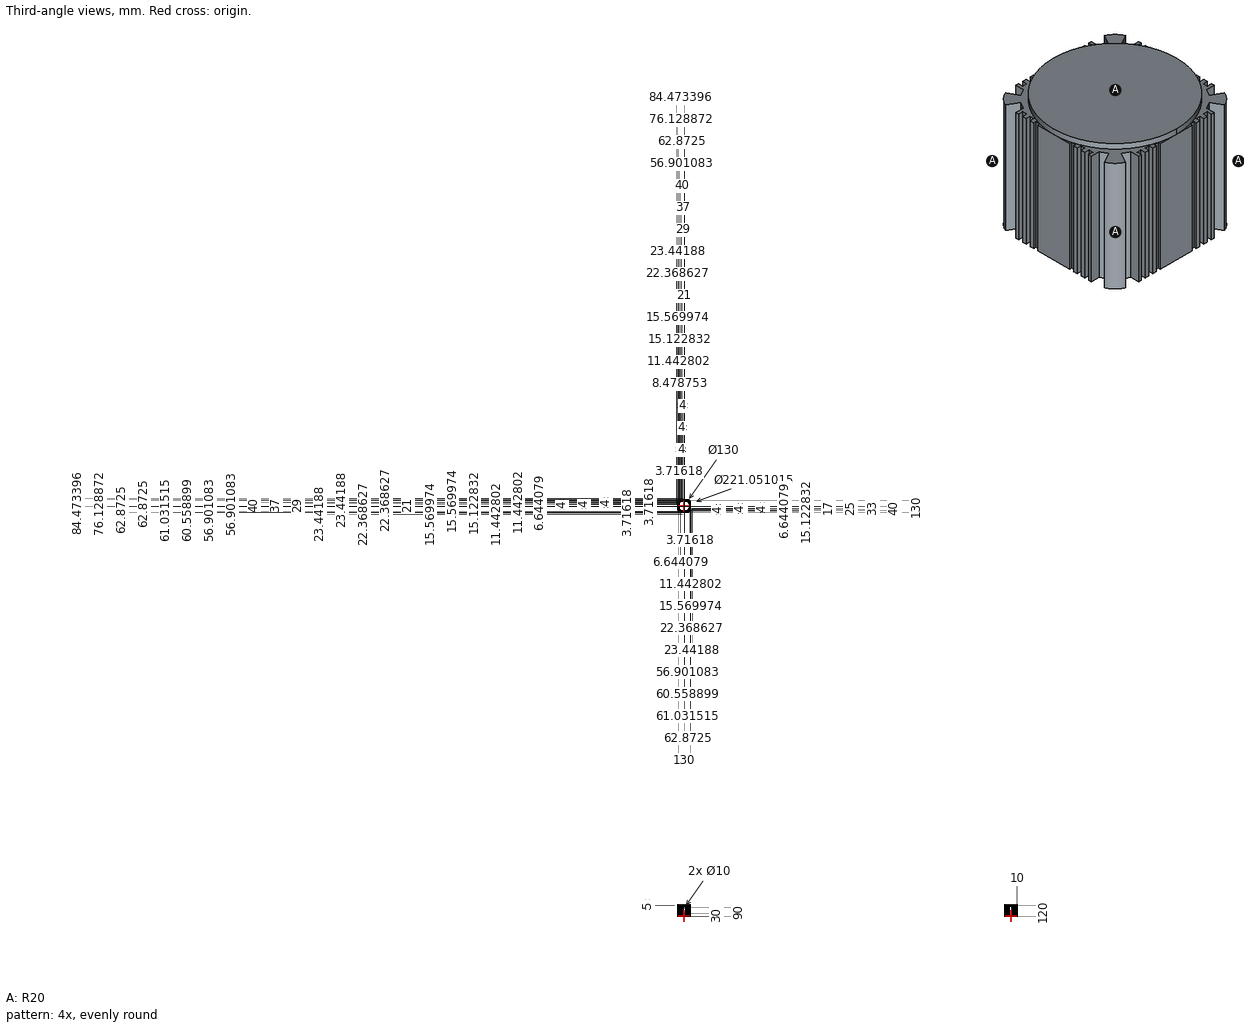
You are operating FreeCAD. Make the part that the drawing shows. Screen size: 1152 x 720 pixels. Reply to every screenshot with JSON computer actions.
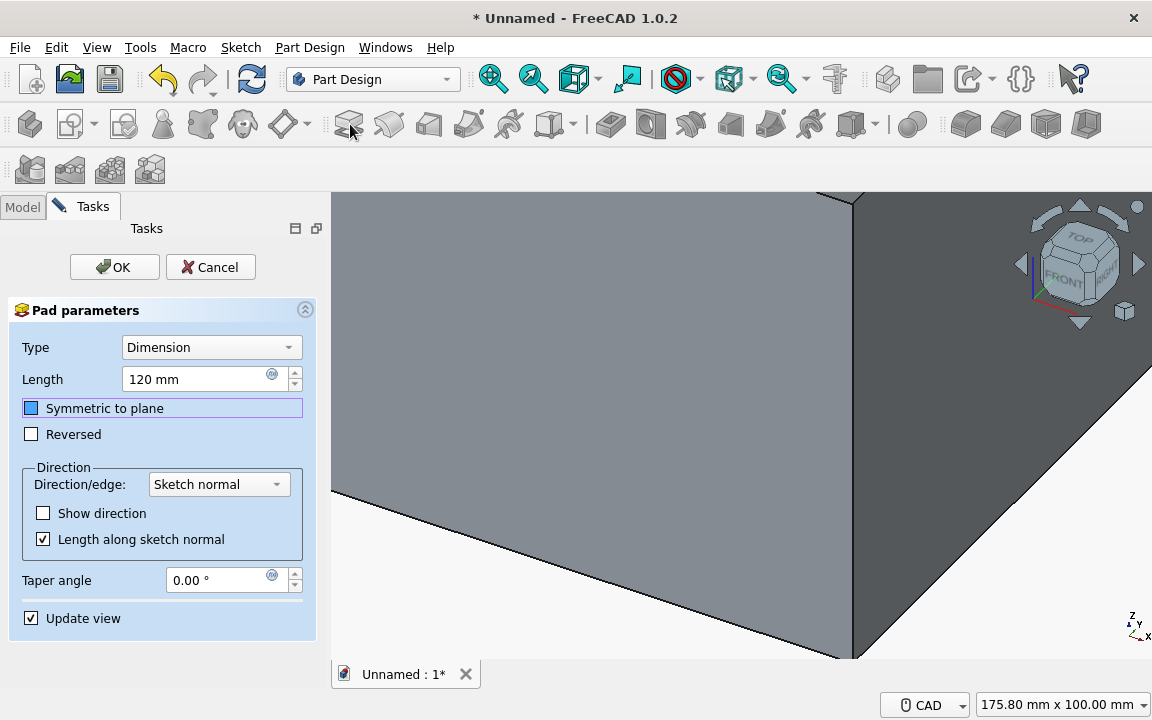
{"action": "left_click", "coordinate": [115, 267]}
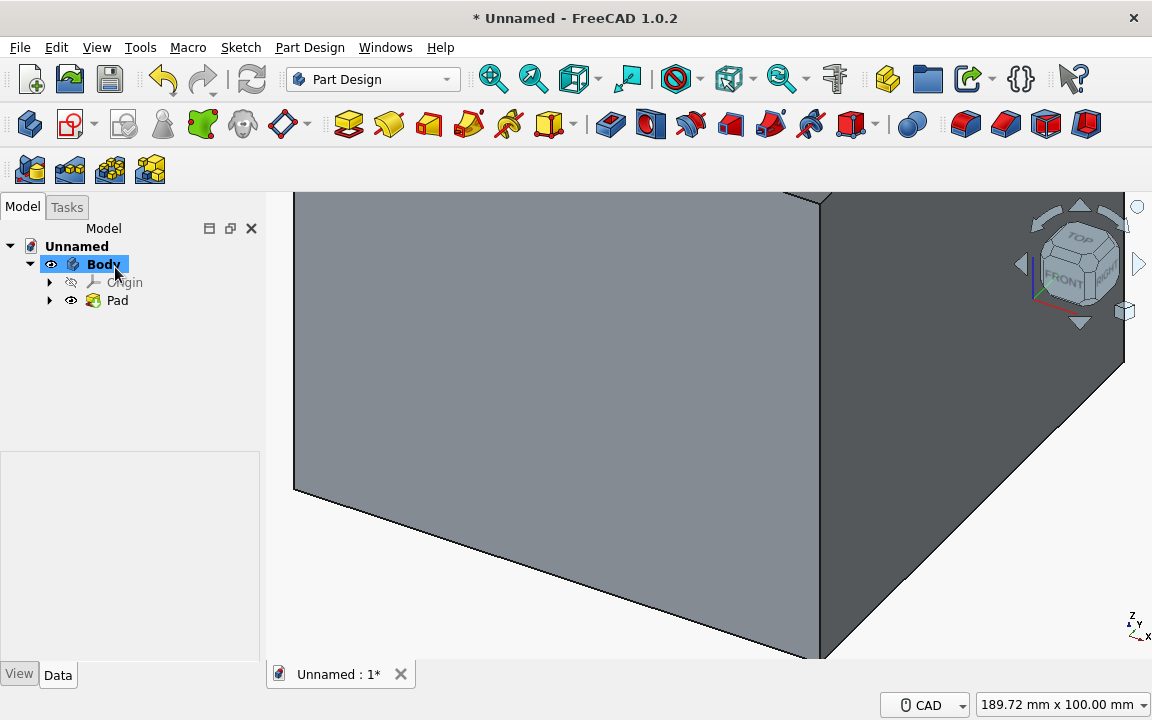
{"action": "left_click", "coordinate": [494, 80]}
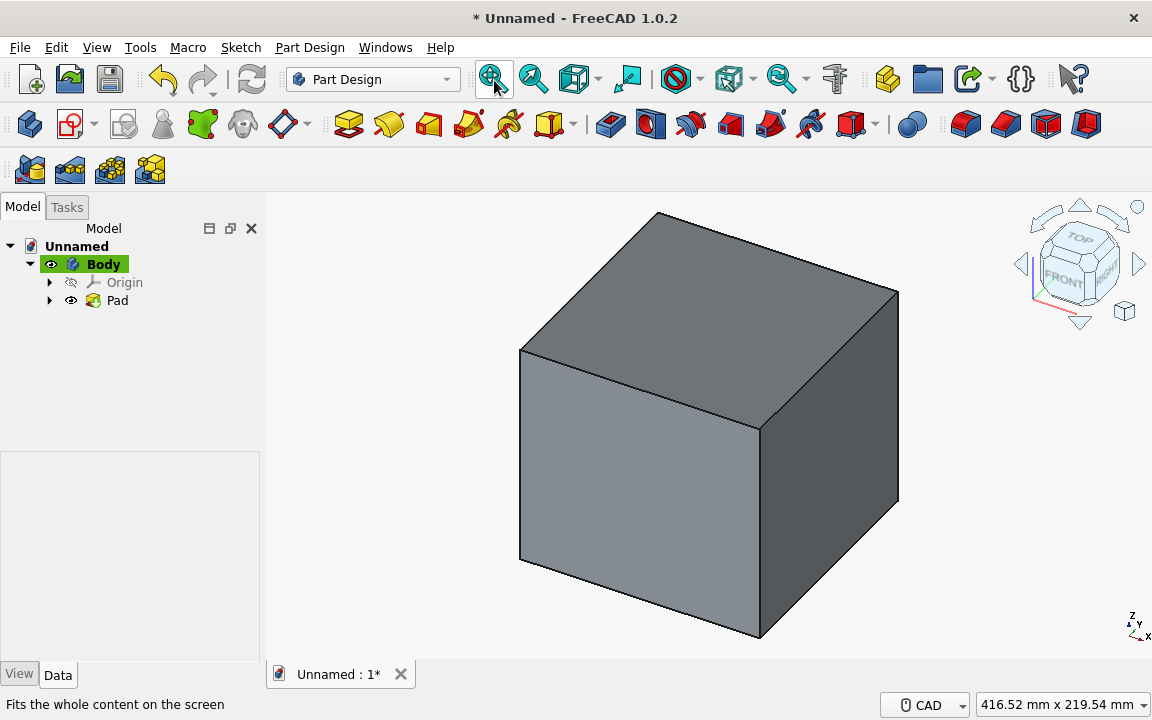
{"action": "left_click", "coordinate": [709, 320]}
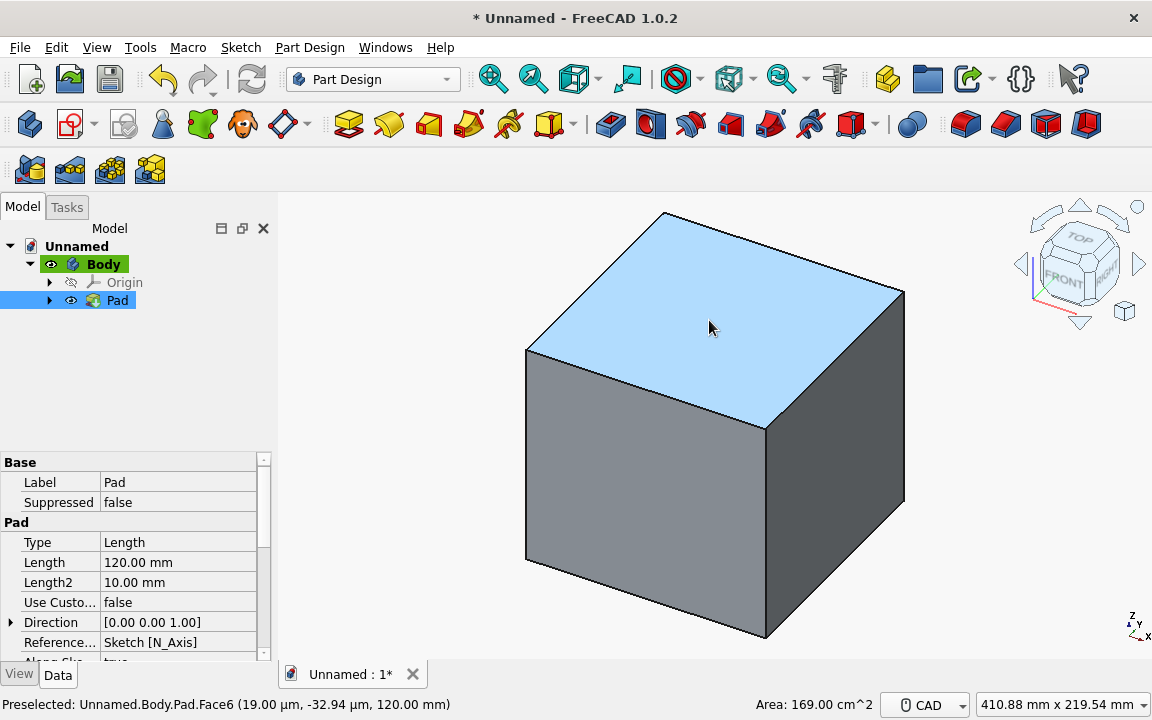
{"action": "left_click", "coordinate": [70, 124]}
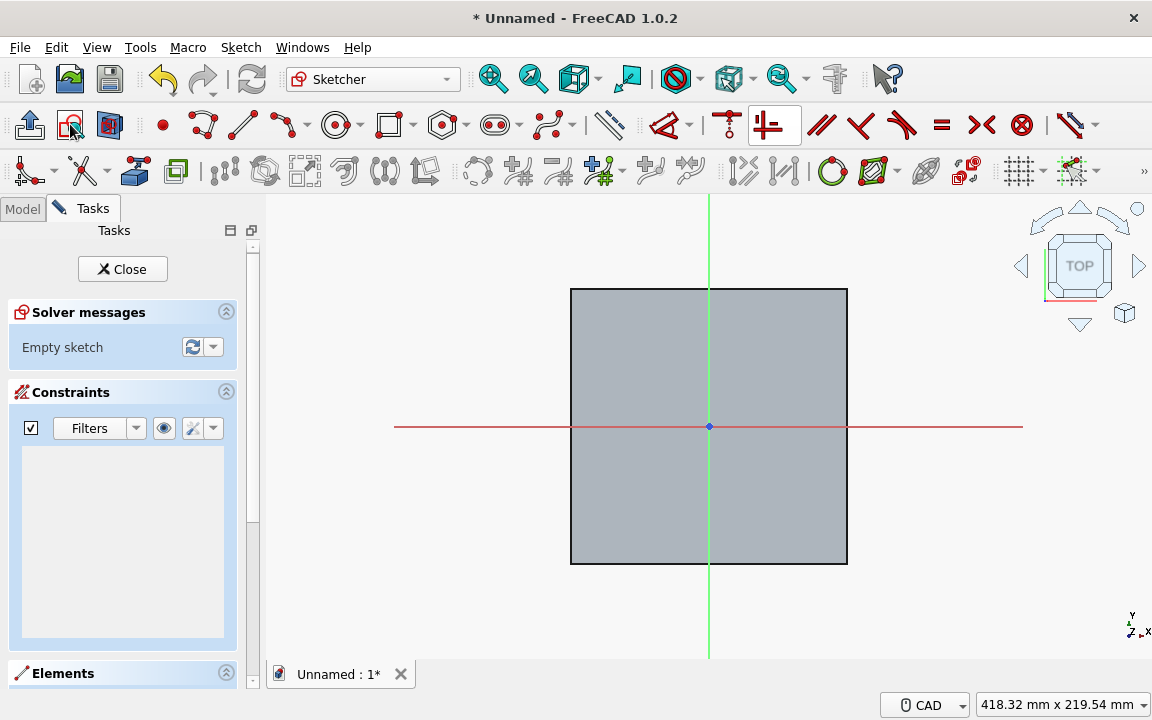
{"action": "scroll", "coordinate": [501, 427], "scroll_direction": "down", "scroll_amount": 2}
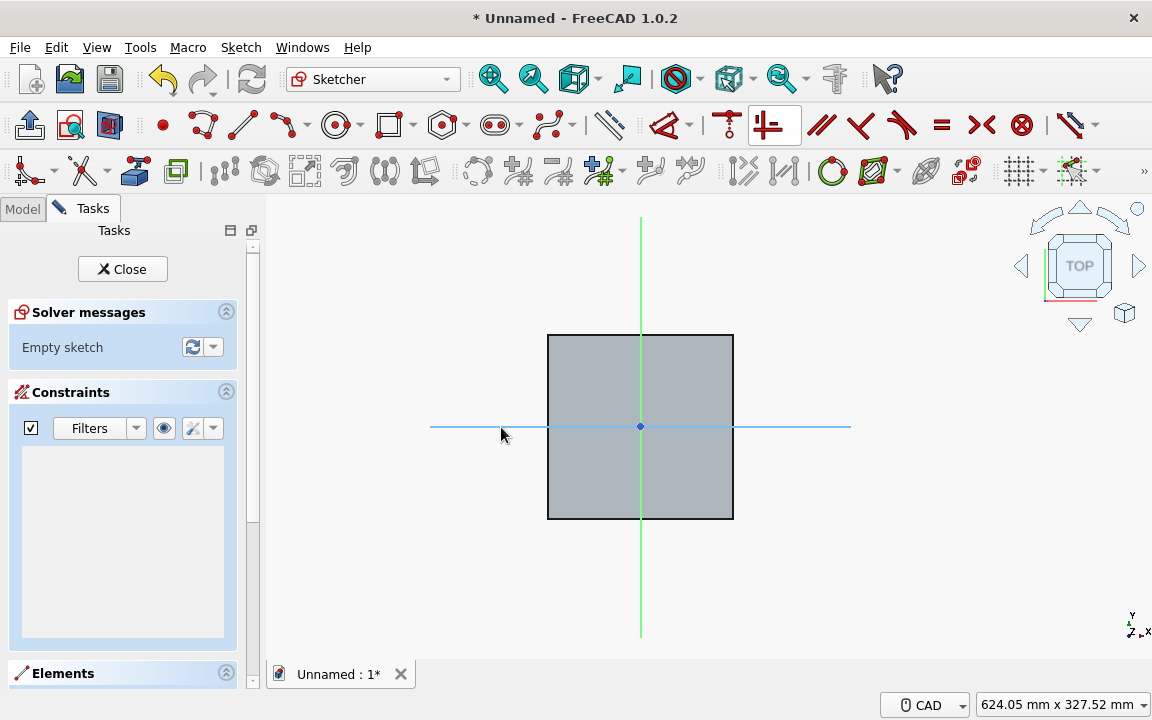
{"action": "key", "text": "g c"}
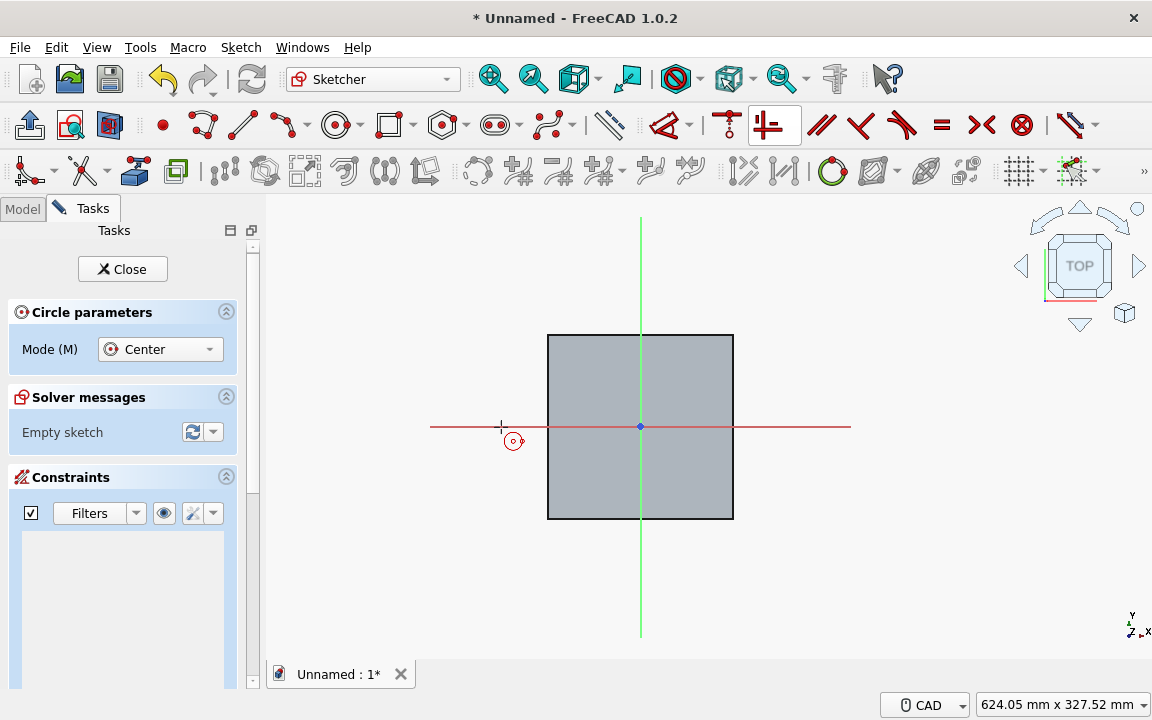
{"action": "left_click", "coordinate": [641, 427]}
{"action": "mouse_move", "coordinate": [751, 316]}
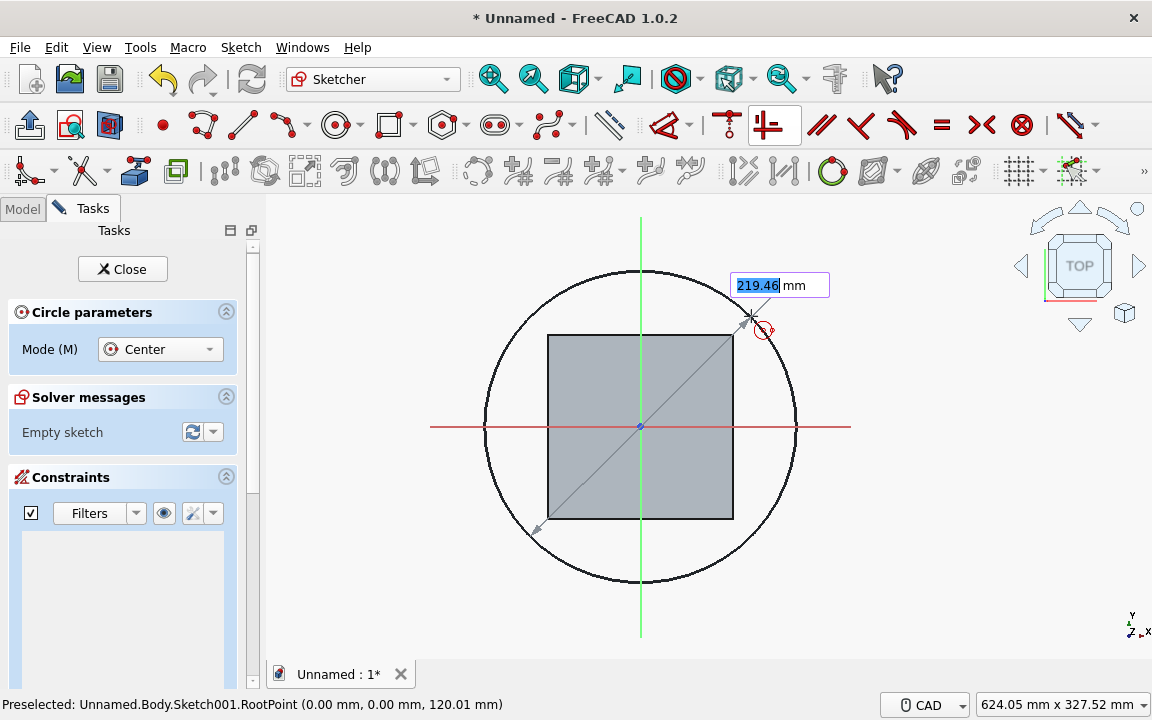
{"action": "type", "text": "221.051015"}
{"action": "key", "text": "Return"}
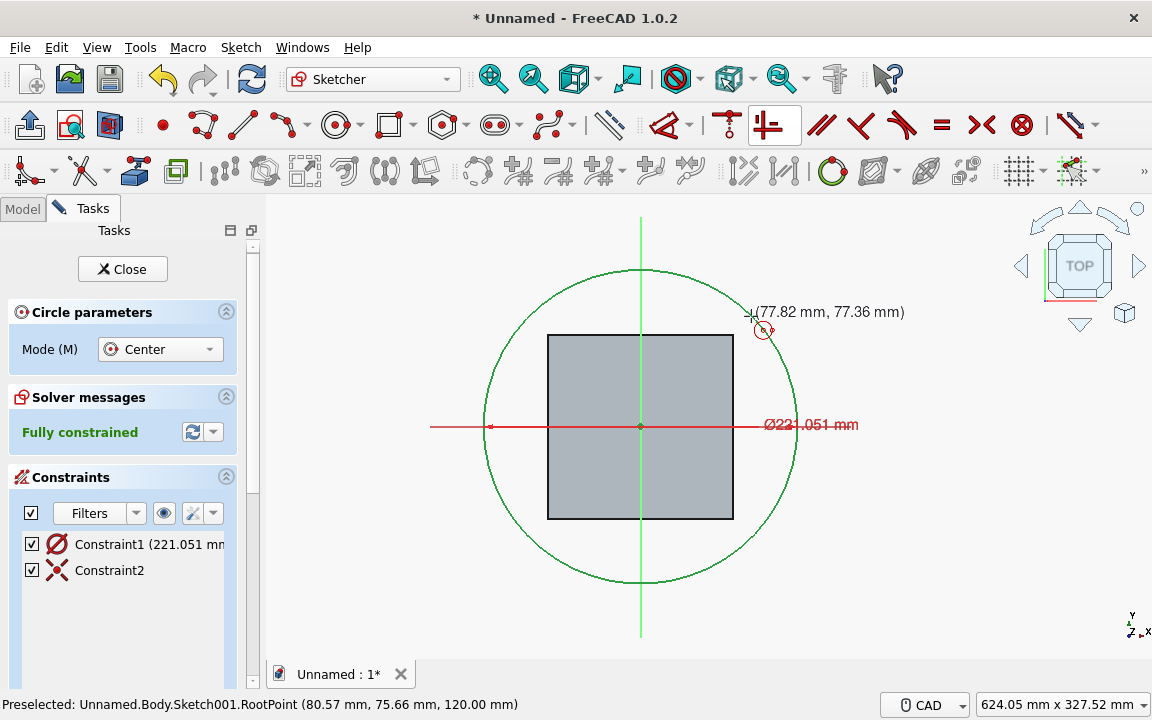
{"action": "left_click", "coordinate": [641, 427]}
{"action": "mouse_move", "coordinate": [706, 362]}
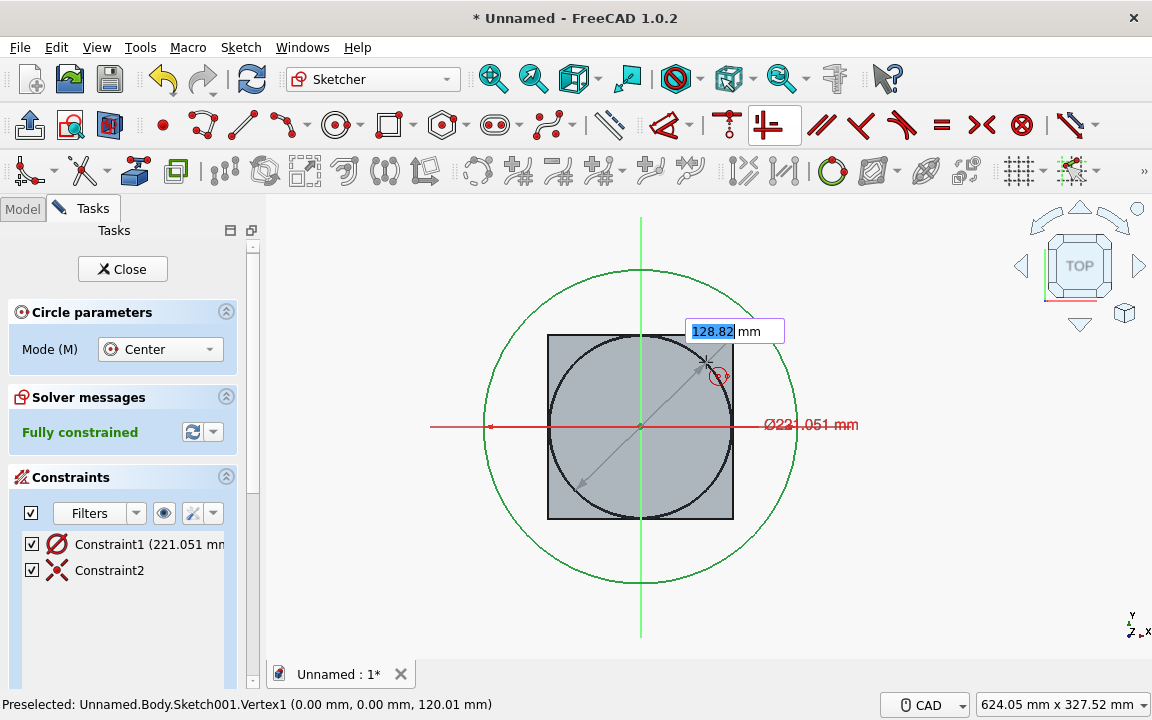
{"action": "type", "text": "130"}
{"action": "key", "text": "Return"}
{"action": "key", "text": "Escape"}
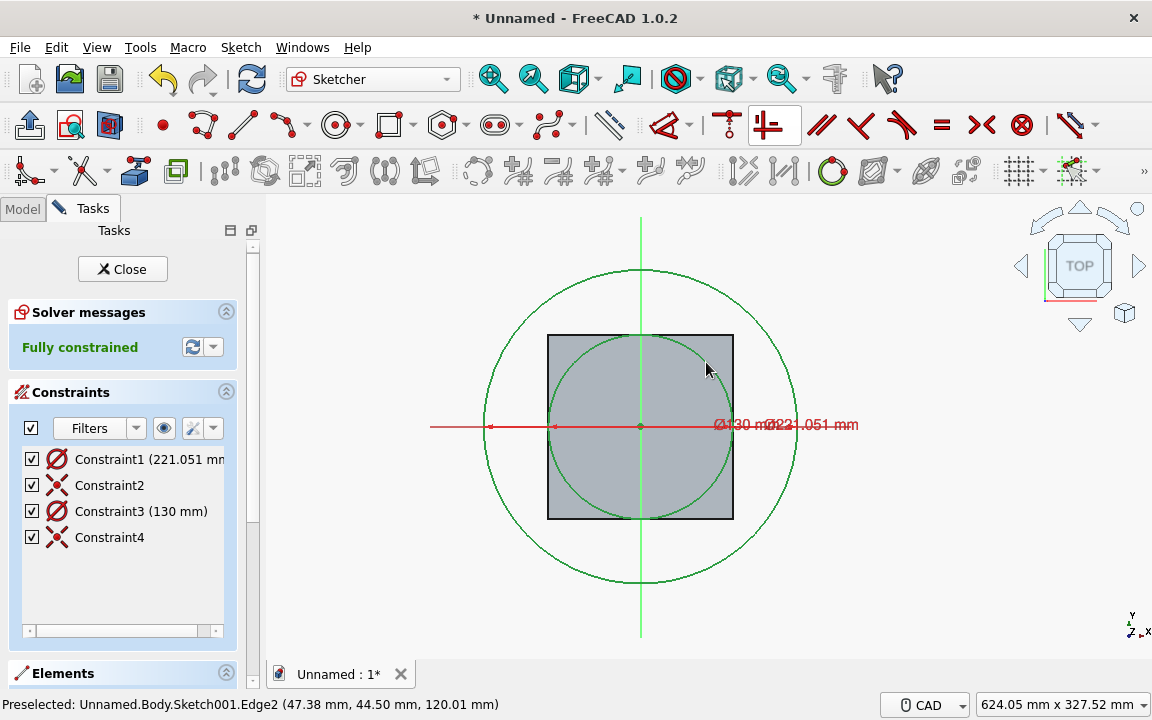
{"action": "left_click", "coordinate": [123, 269]}